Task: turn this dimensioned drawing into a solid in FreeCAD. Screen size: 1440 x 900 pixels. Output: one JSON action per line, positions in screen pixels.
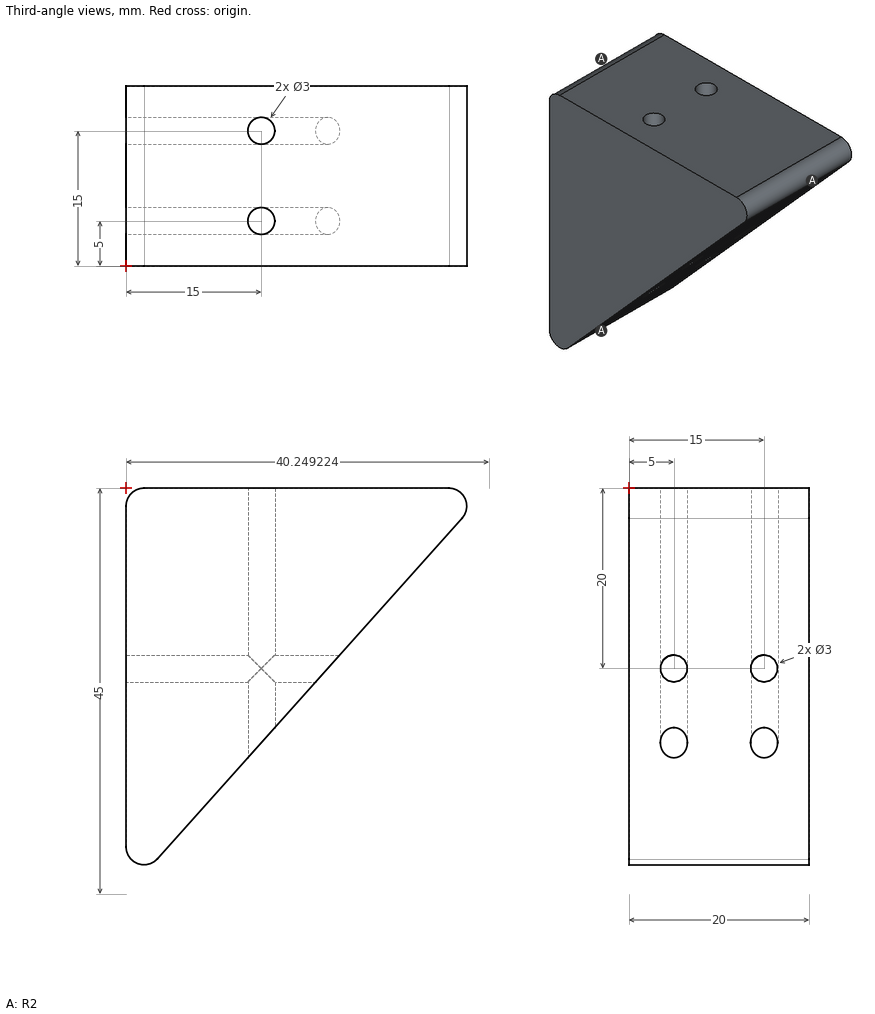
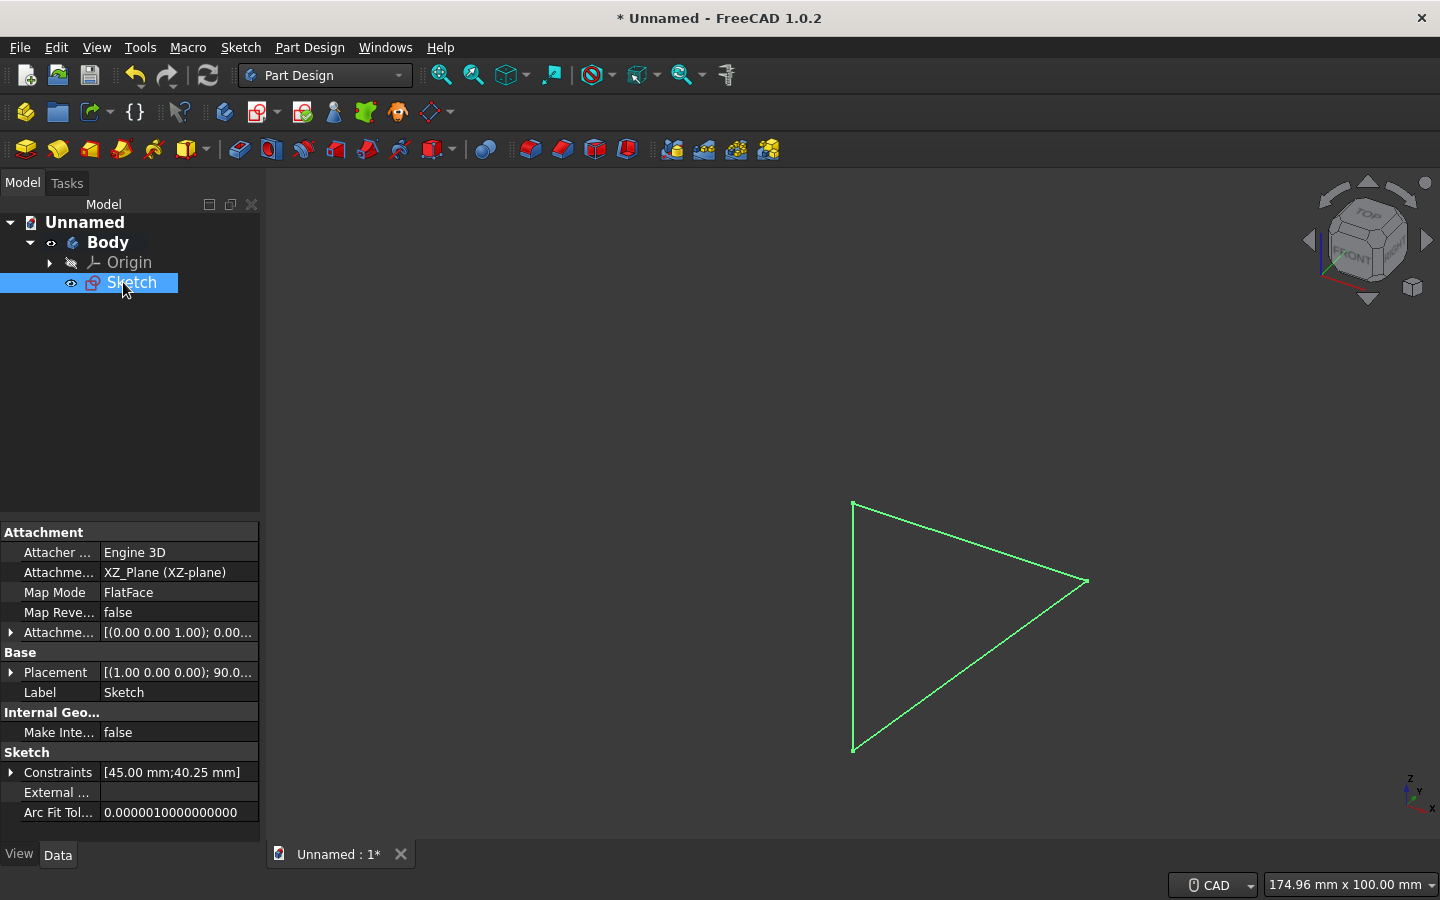
{"action": "left_click", "coordinate": [26, 150]}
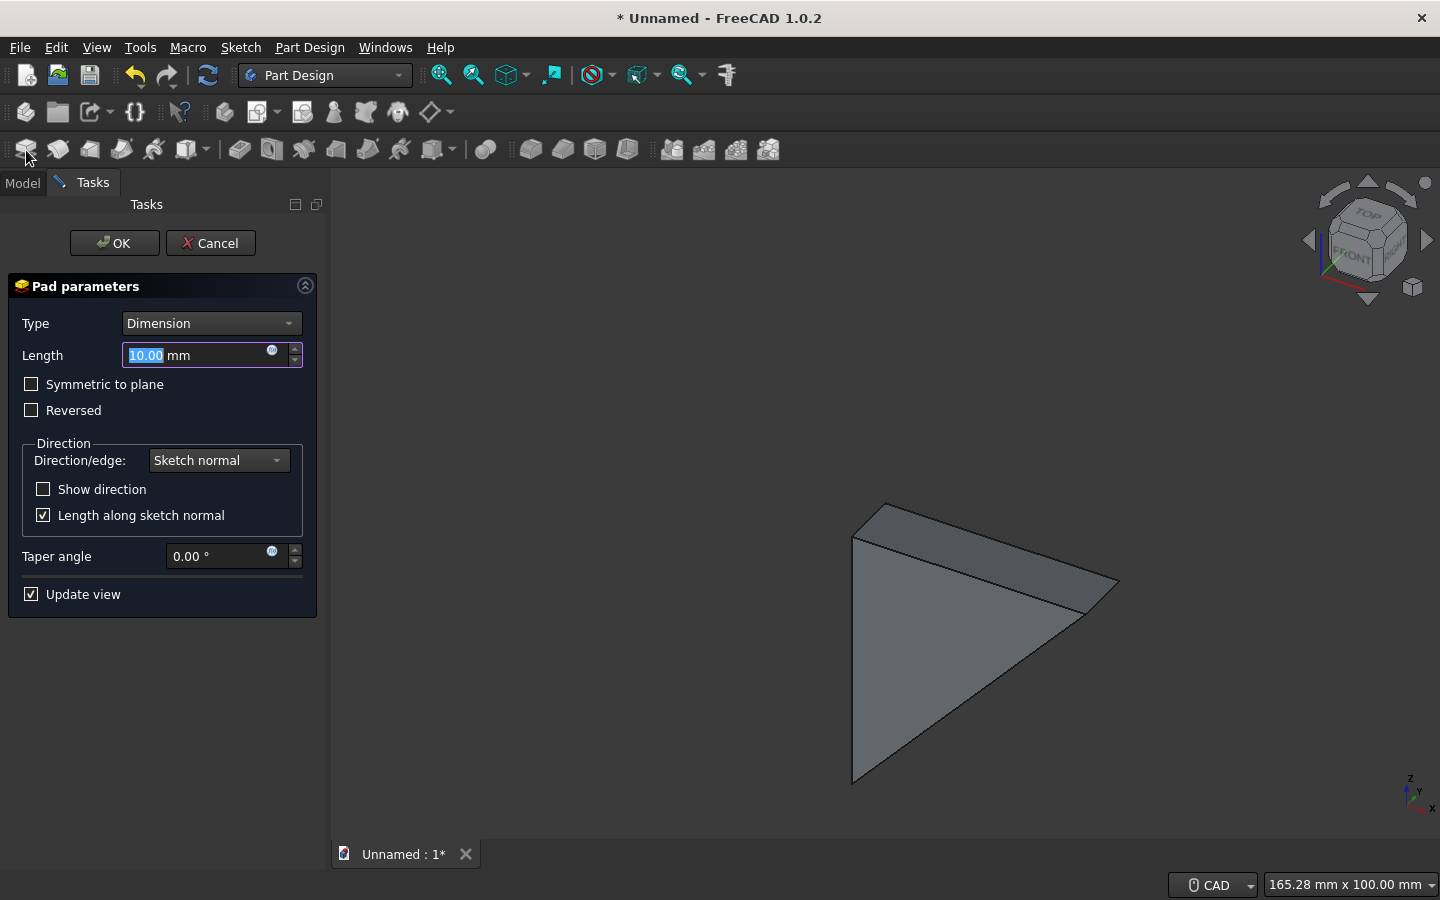
{"action": "type", "text": "20"}
{"action": "key", "text": "Tab"}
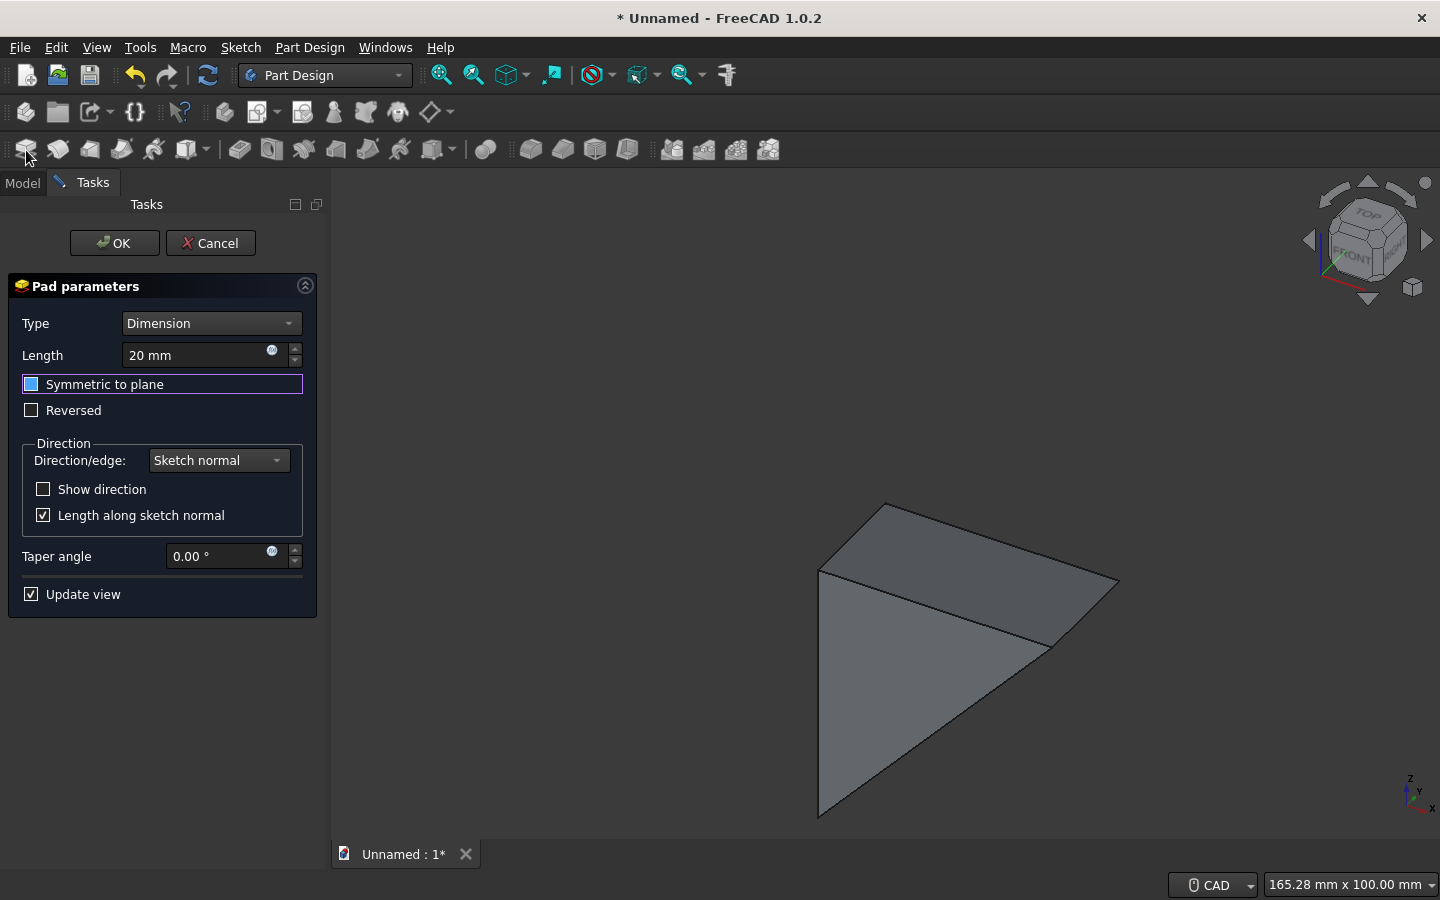
{"action": "left_click", "coordinate": [30, 410]}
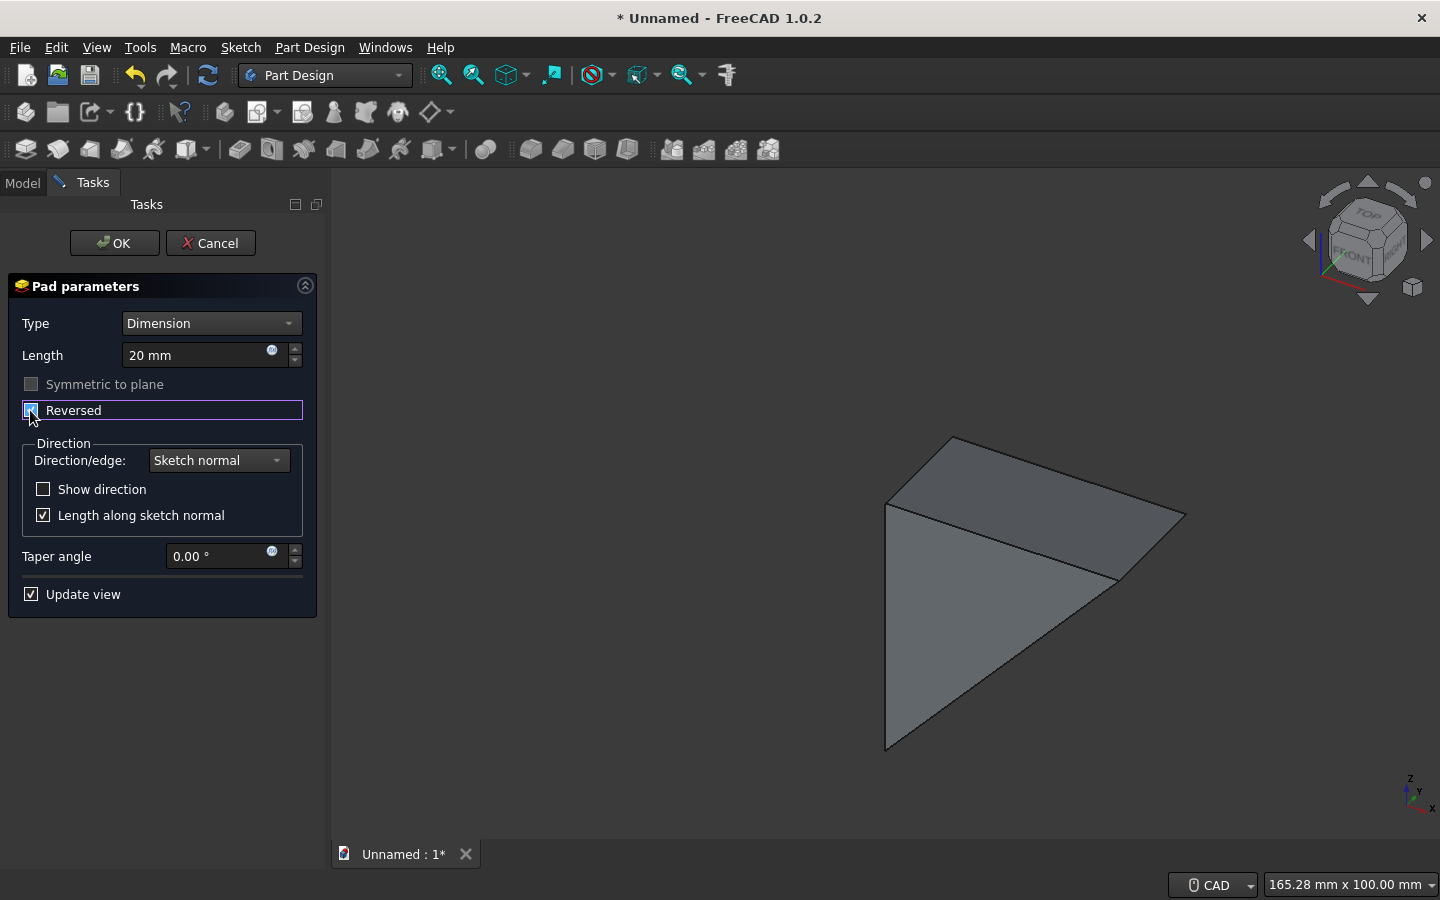
{"action": "left_click", "coordinate": [115, 243]}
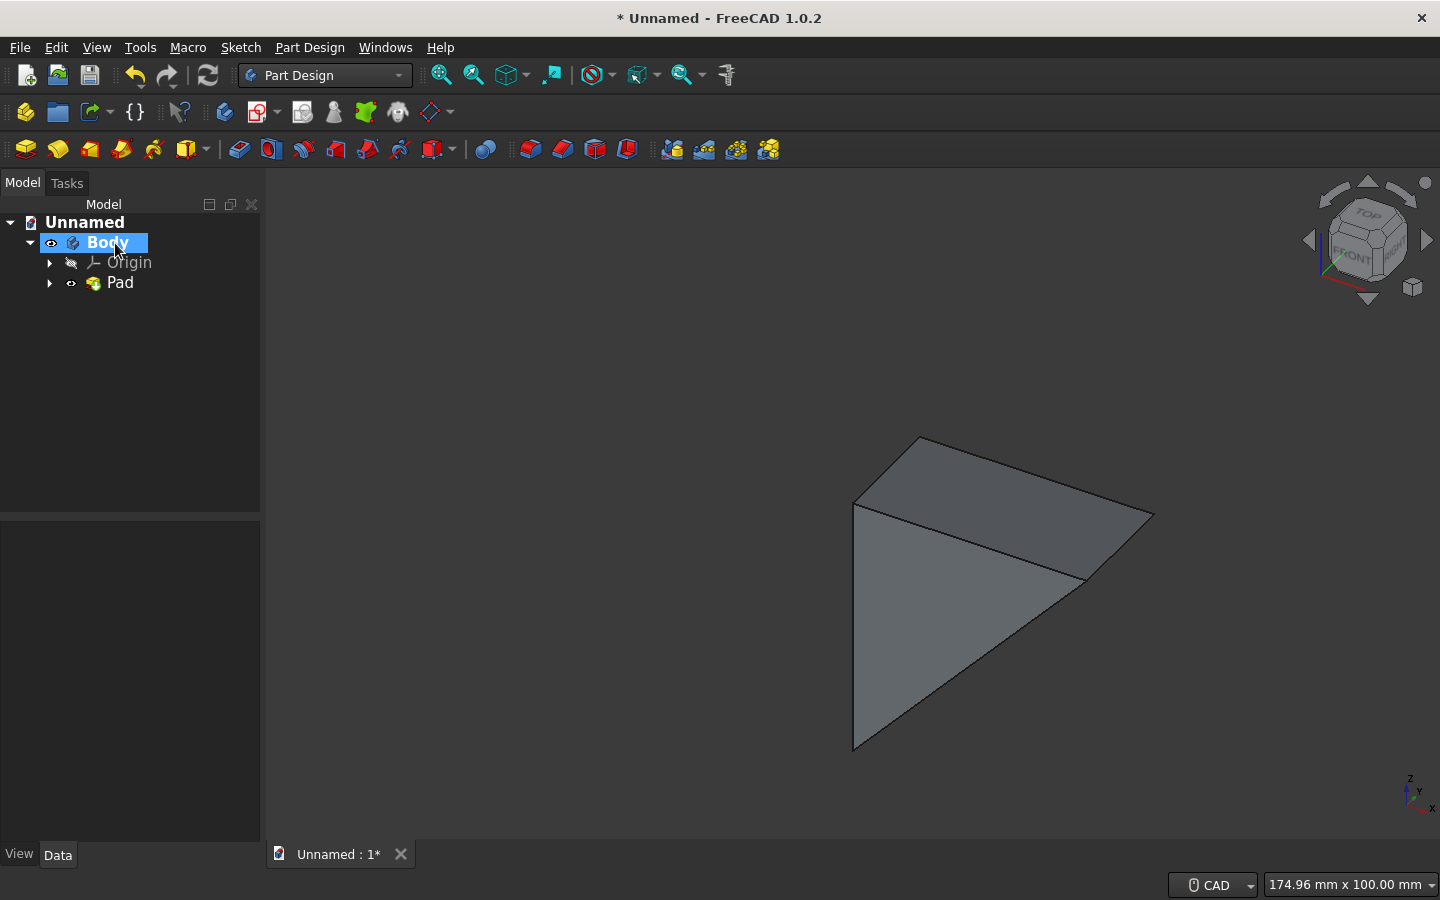
{"action": "left_click", "coordinate": [1120, 547]}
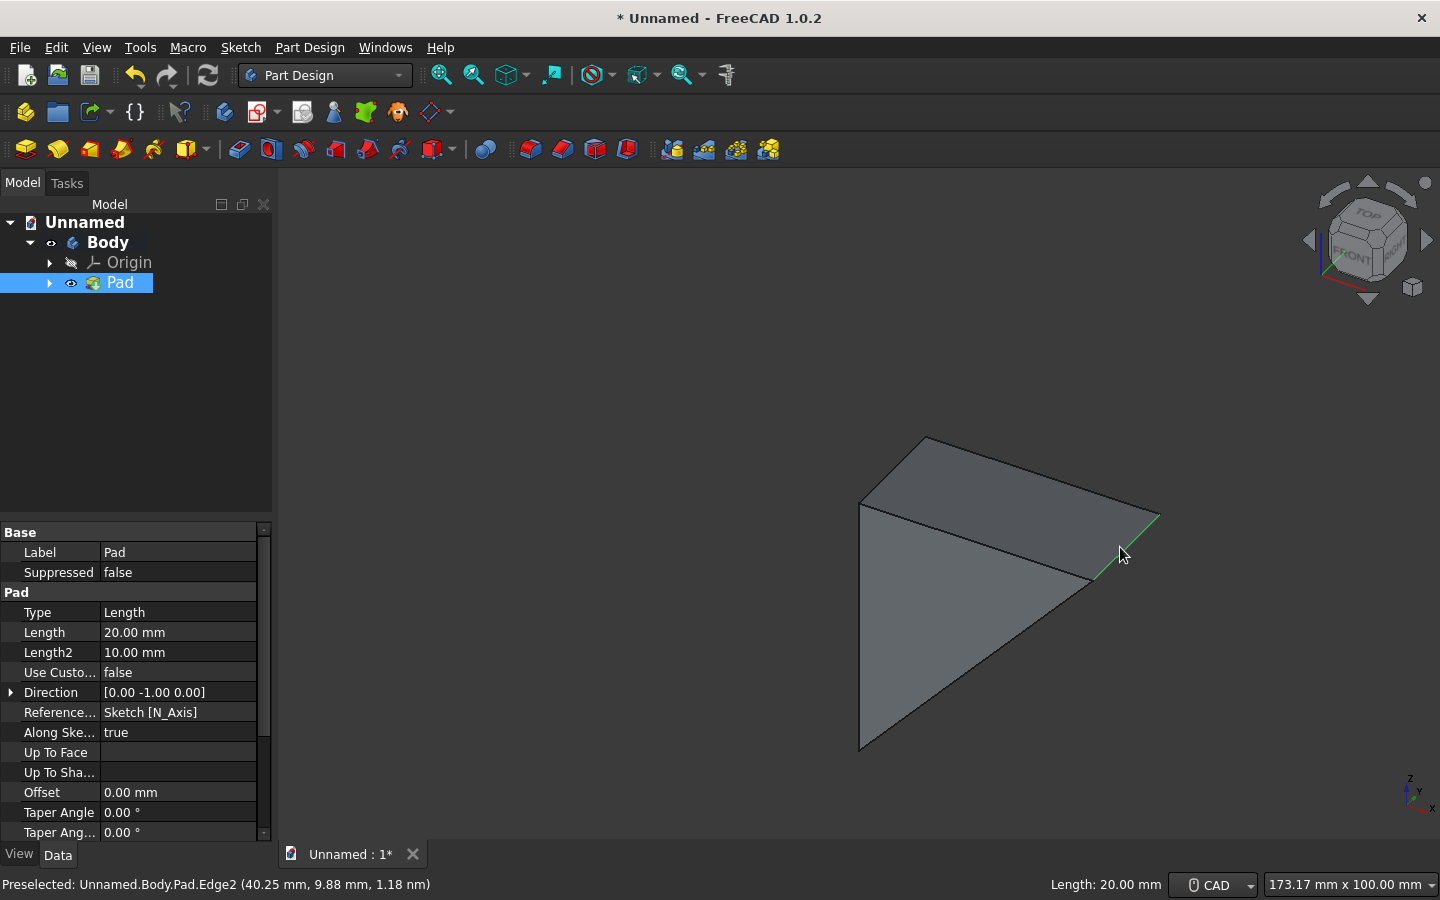
{"action": "key", "text": "0"}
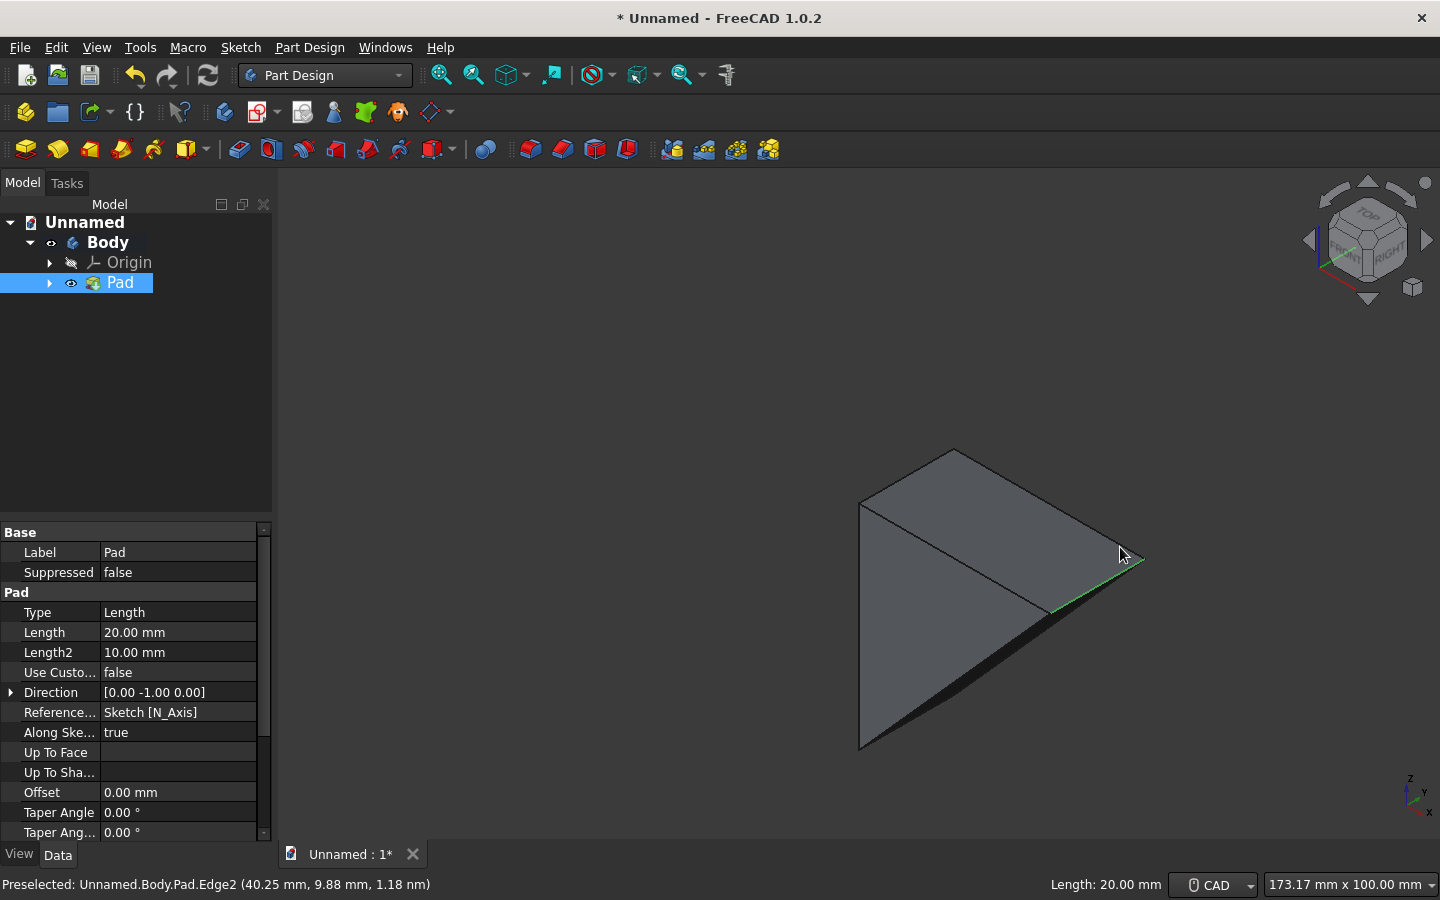
{"action": "key", "text": "v f"}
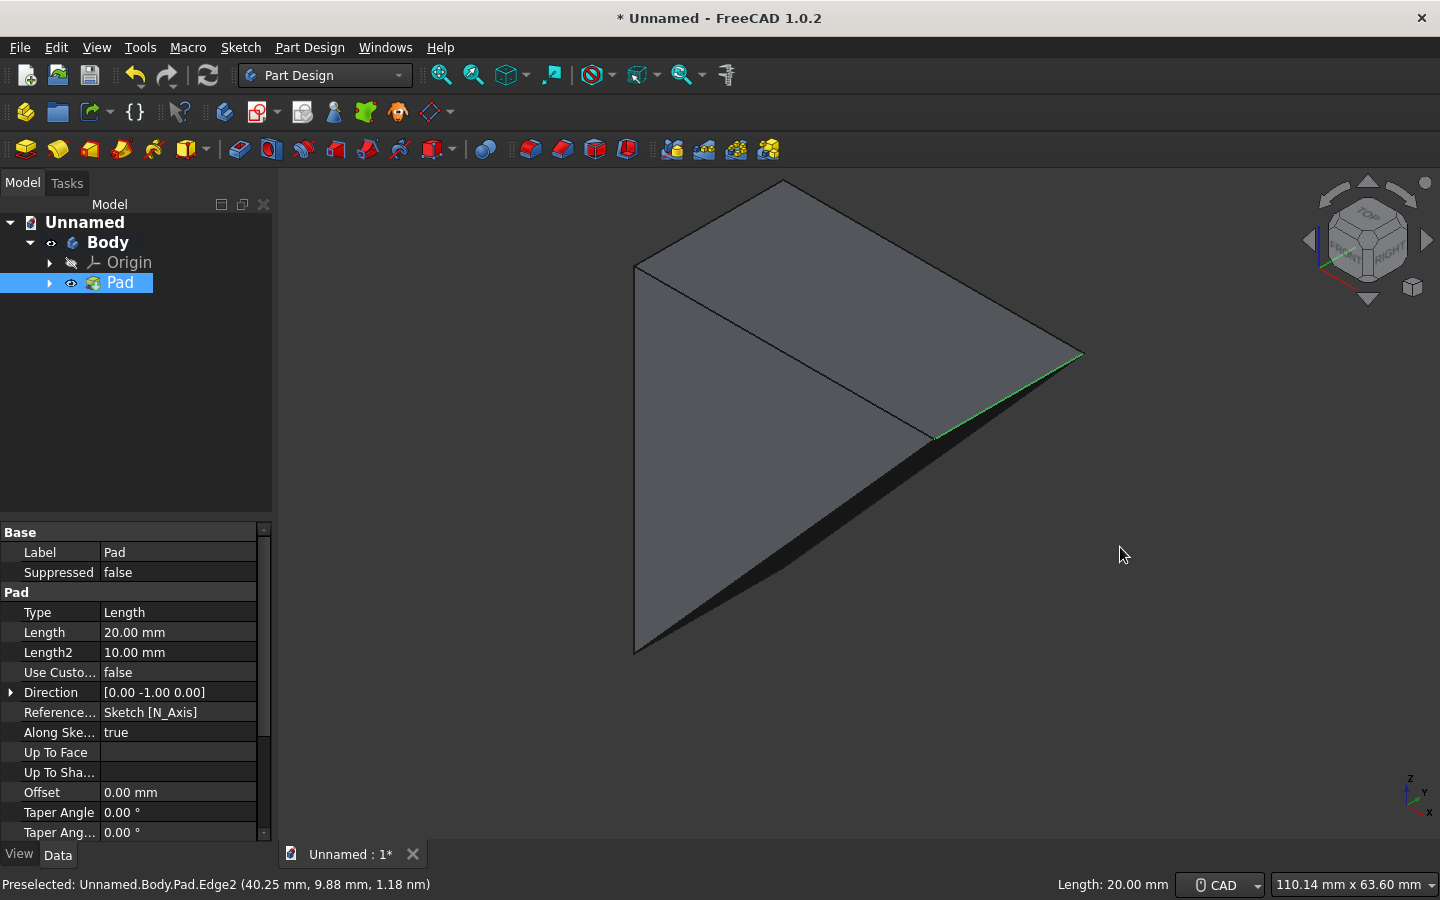
{"action": "key", "text": "2"}